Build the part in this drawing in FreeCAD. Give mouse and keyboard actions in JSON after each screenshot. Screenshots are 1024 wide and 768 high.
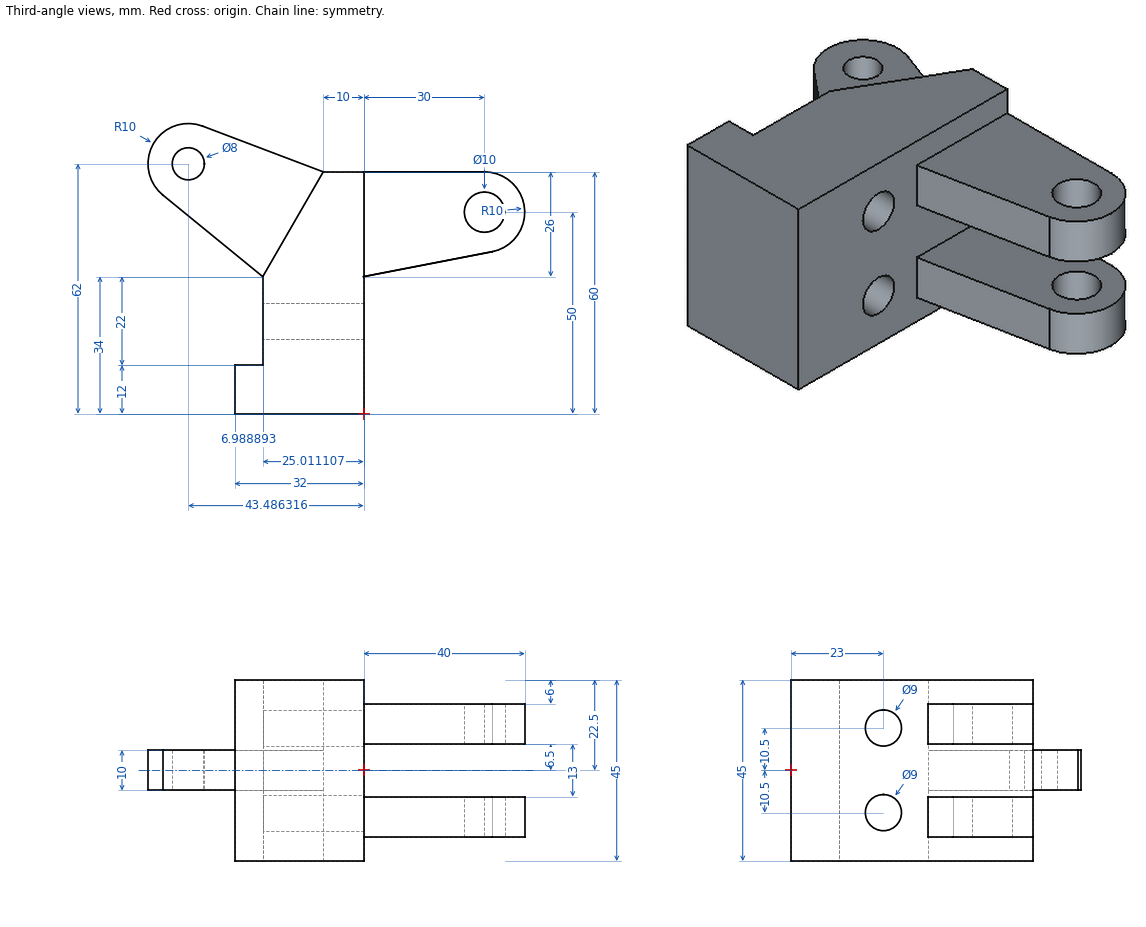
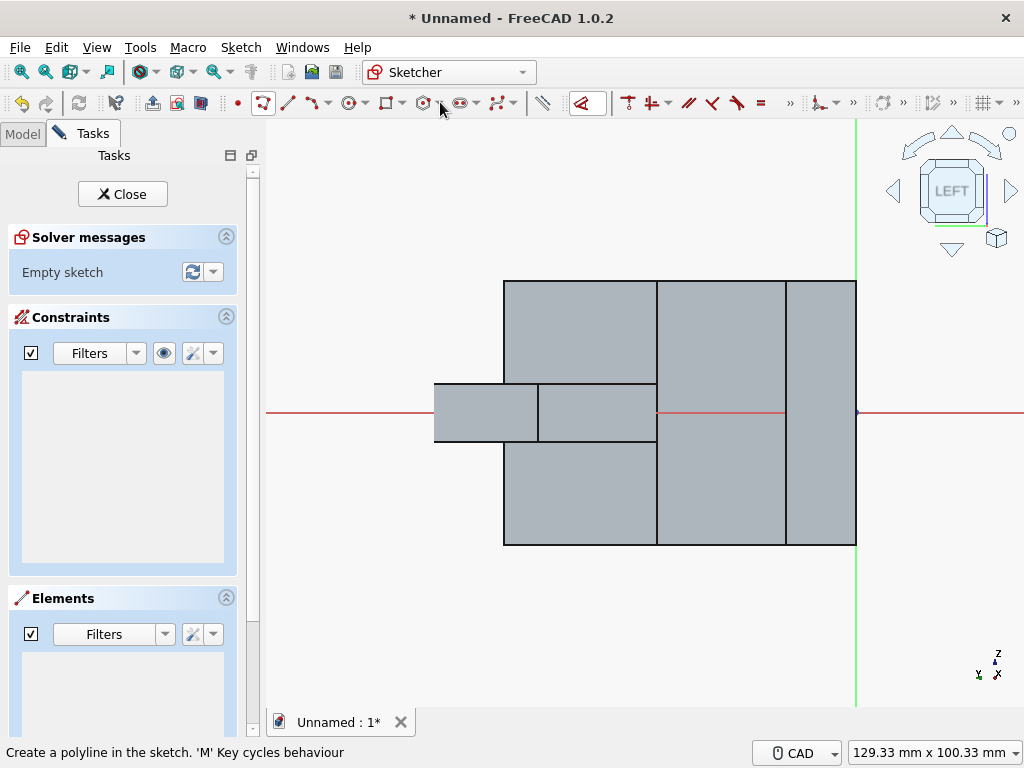
{"action": "scroll", "coordinate": [744, 342], "scroll_direction": "up", "scroll_amount": 10}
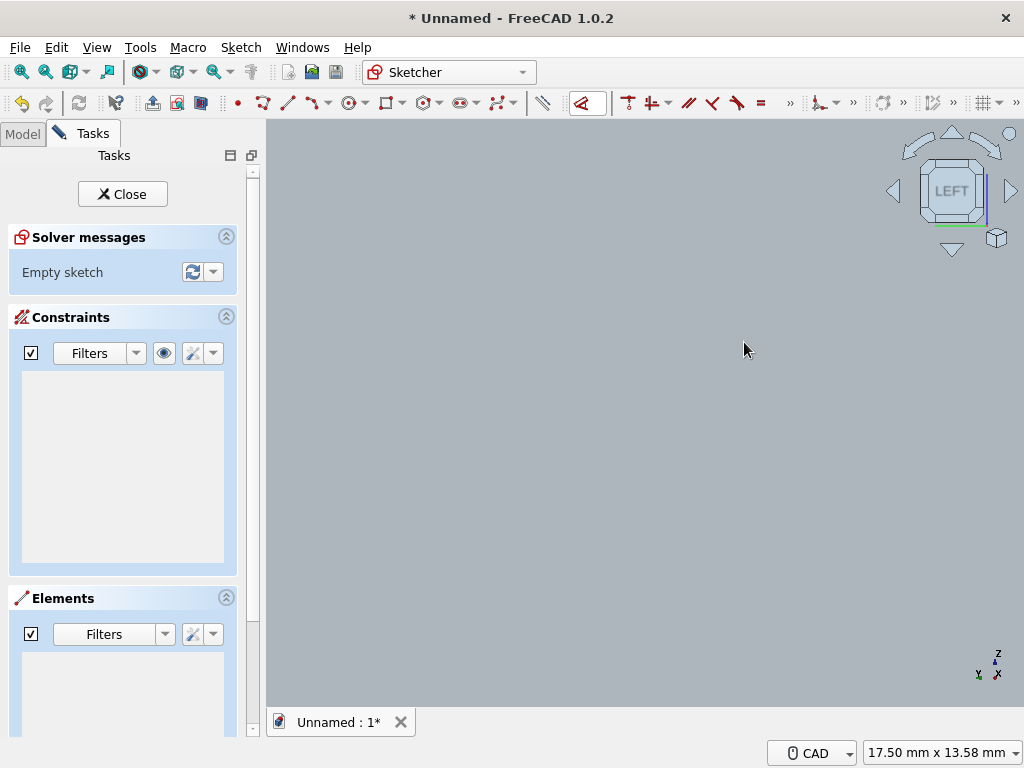
{"action": "key", "text": "g c"}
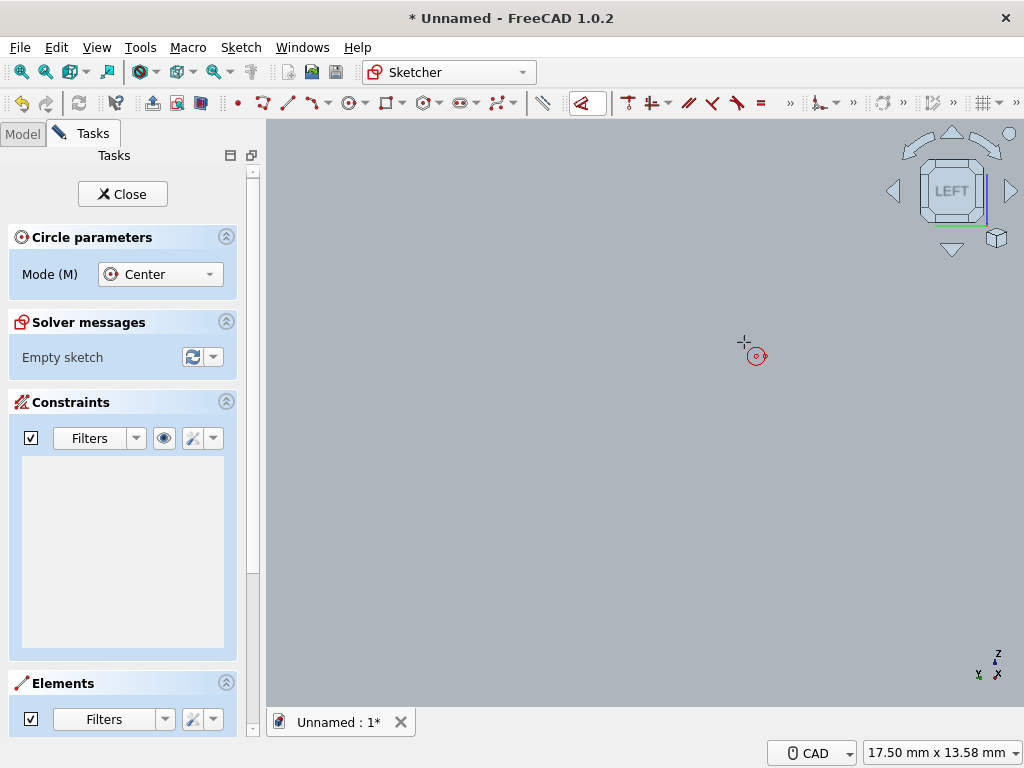
{"action": "left_click", "coordinate": [571, 409]}
{"action": "mouse_move", "coordinate": [709, 272]}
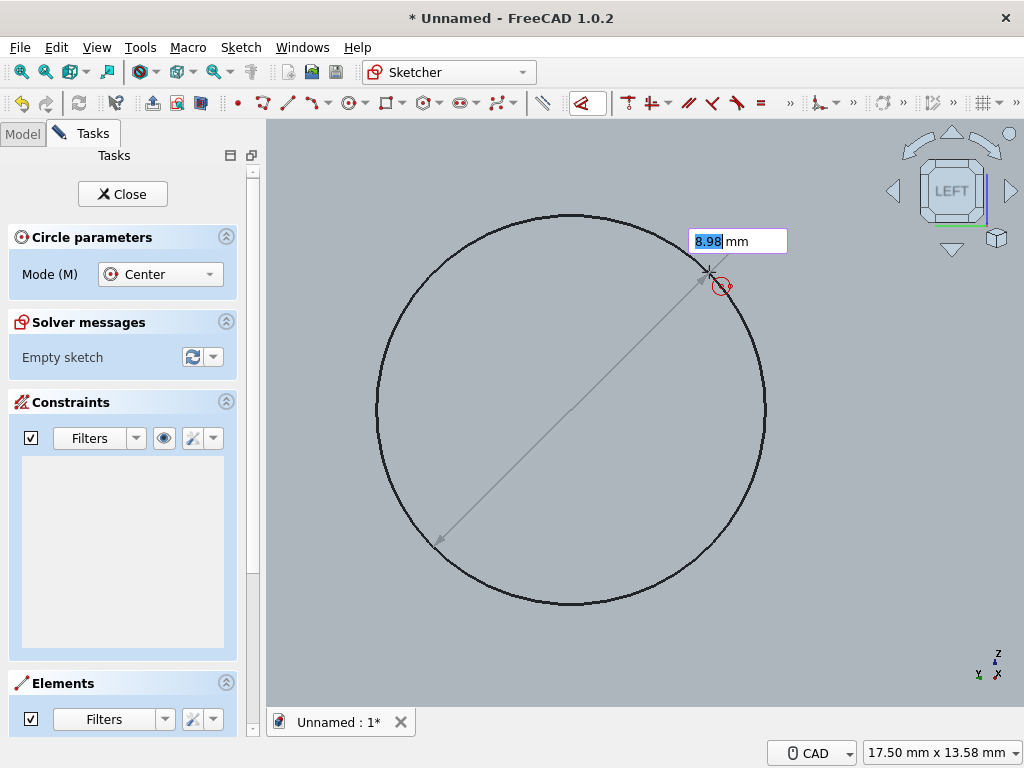
{"action": "type", "text": "9"}
{"action": "key", "text": "Return"}
{"action": "key", "text": "Escape"}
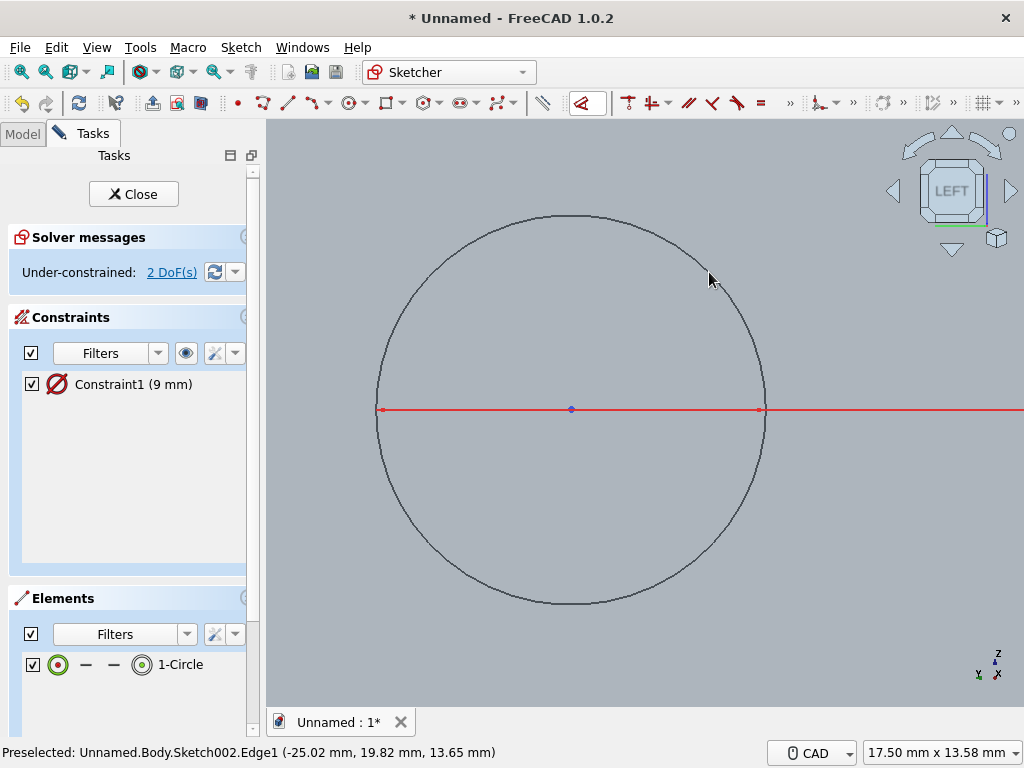
{"action": "left_click", "coordinate": [571, 410]}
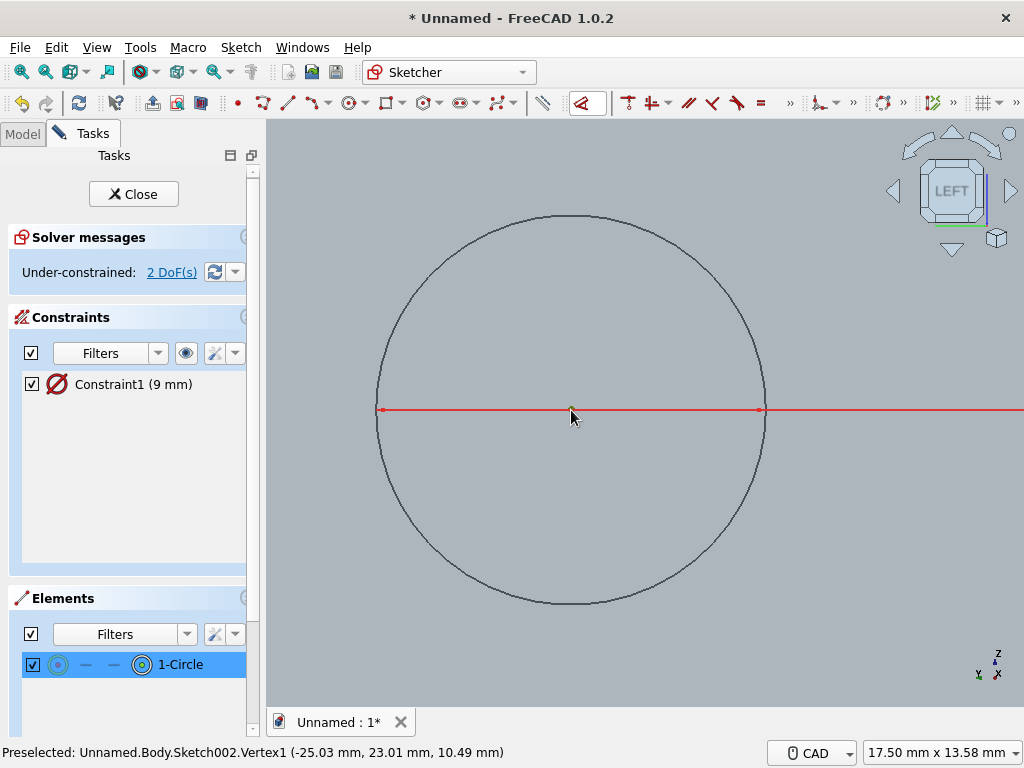
{"action": "key", "text": "l"}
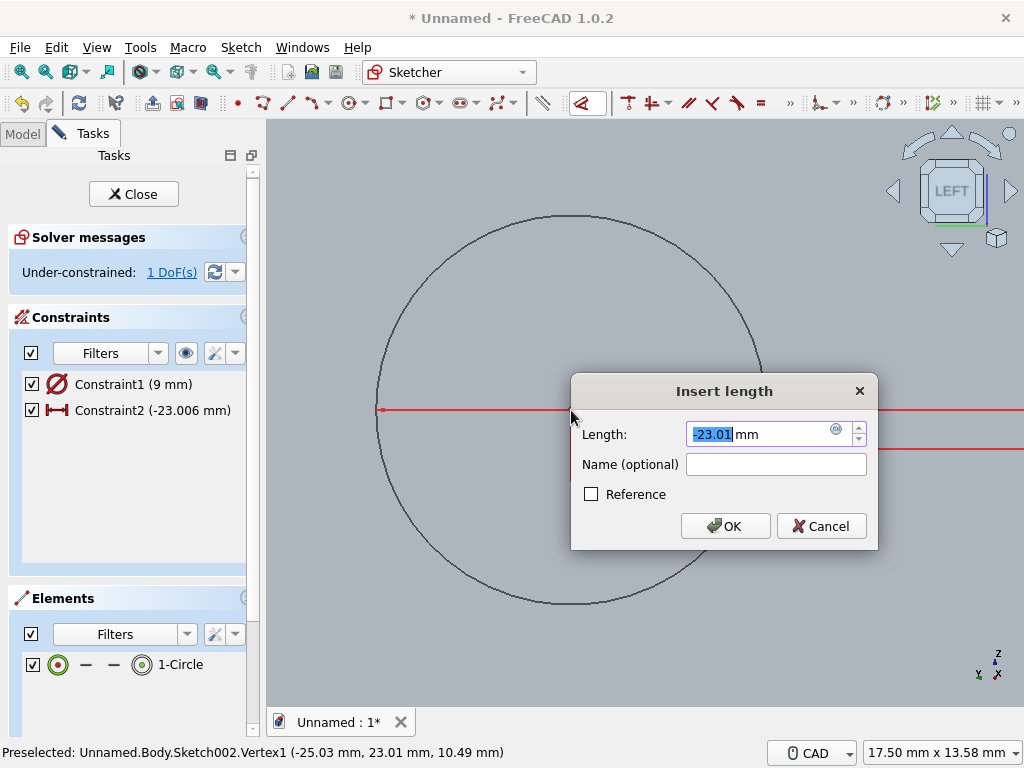
{"action": "type", "text": "-23"}
{"action": "key", "text": "Return"}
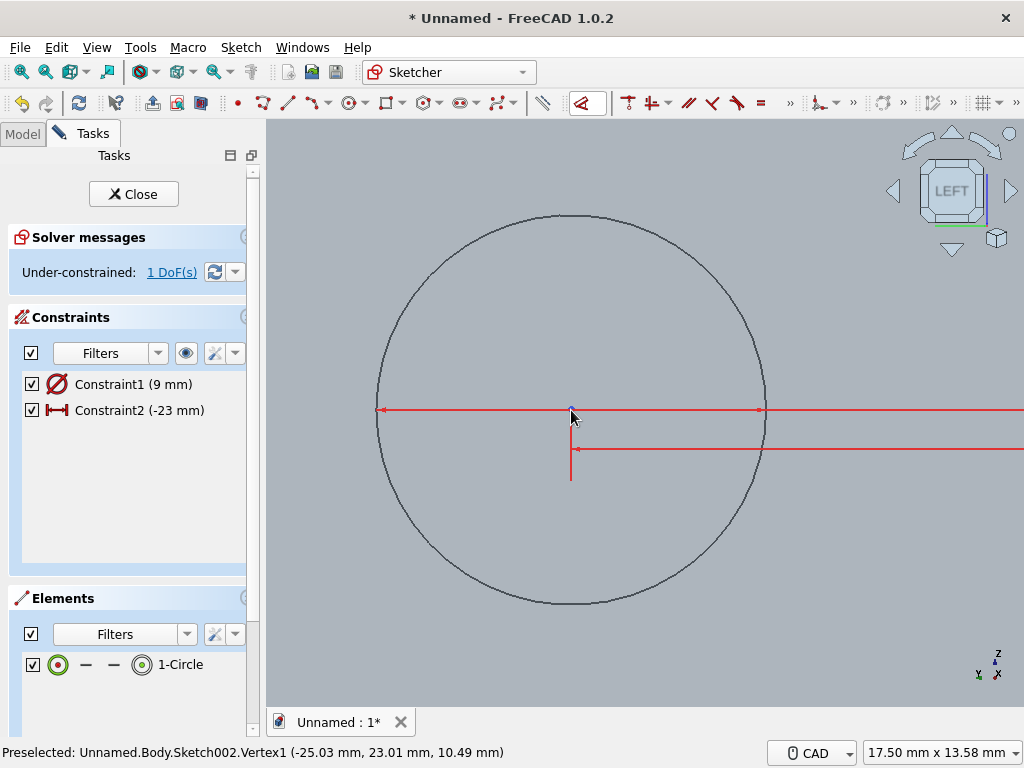
{"action": "left_click", "coordinate": [571, 410]}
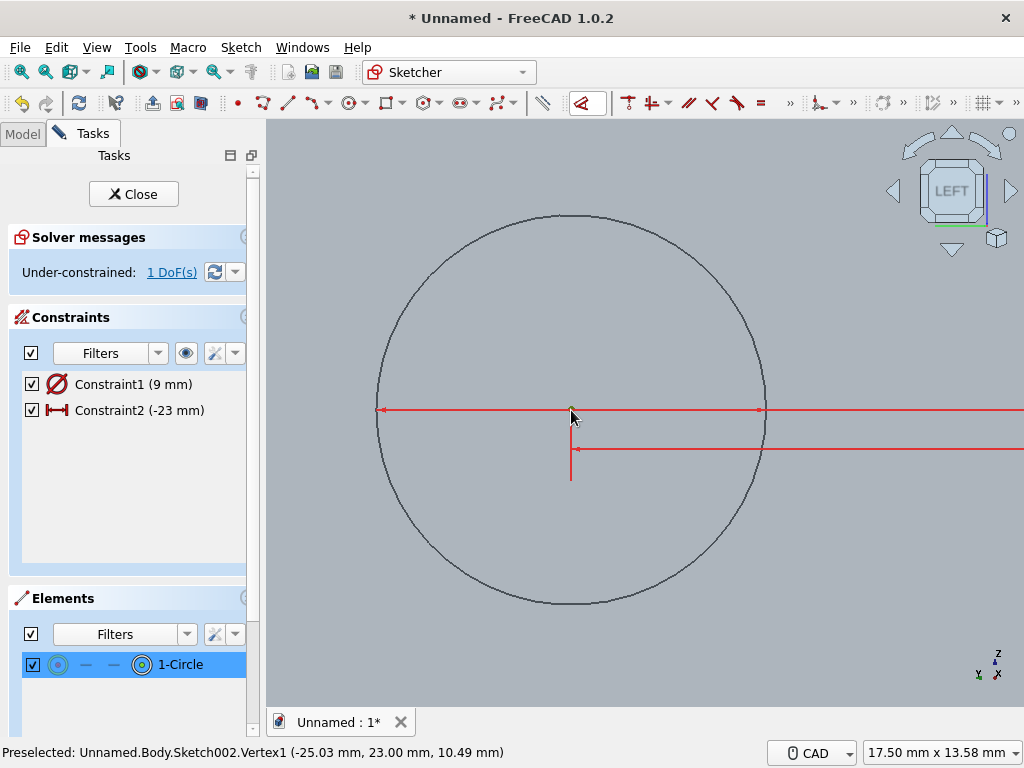
{"action": "key", "text": "i"}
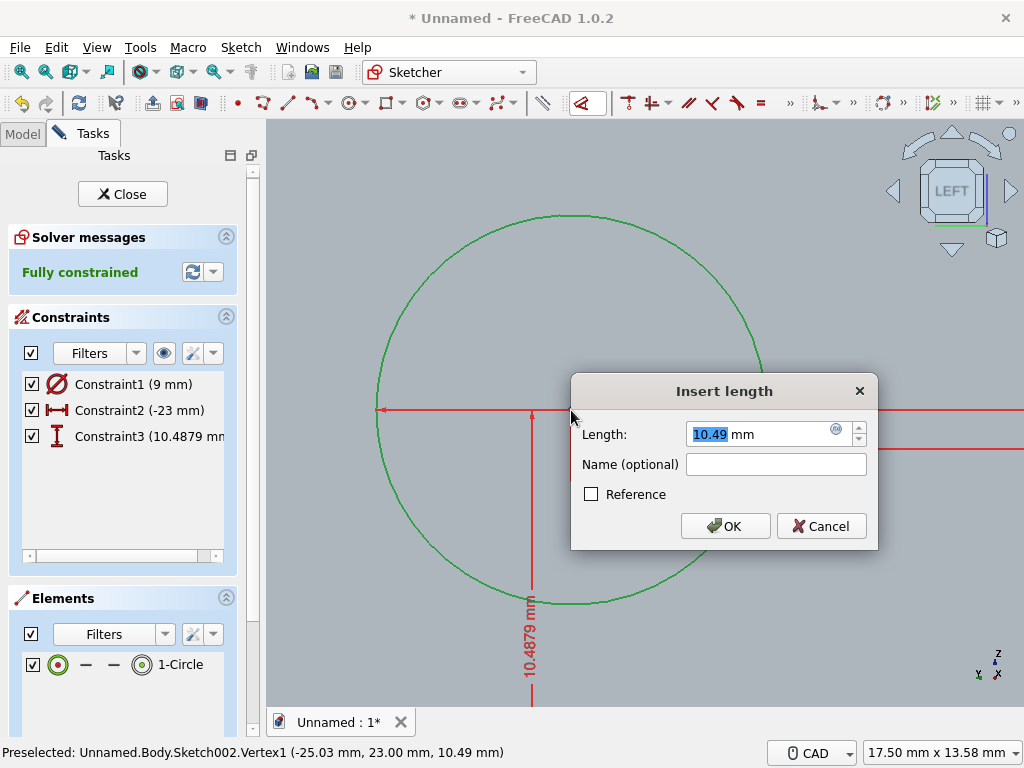
{"action": "type", "text": "10.5"}
{"action": "key", "text": "Return"}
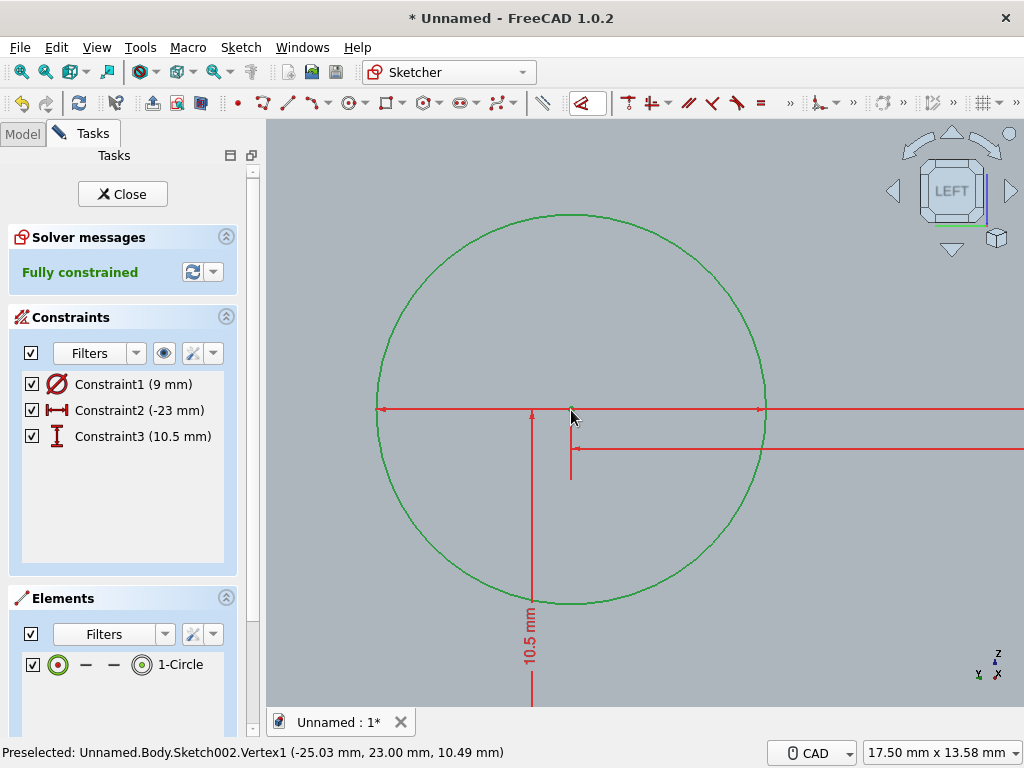
{"action": "left_click", "coordinate": [123, 194]}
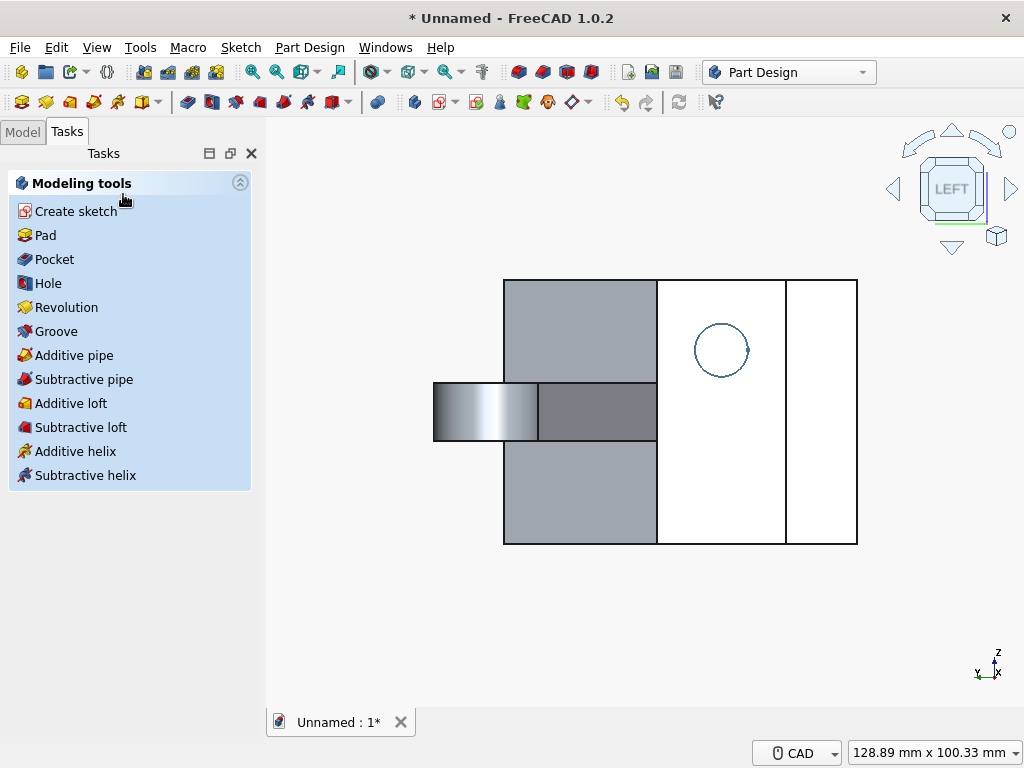
{"action": "left_click", "coordinate": [188, 102]}